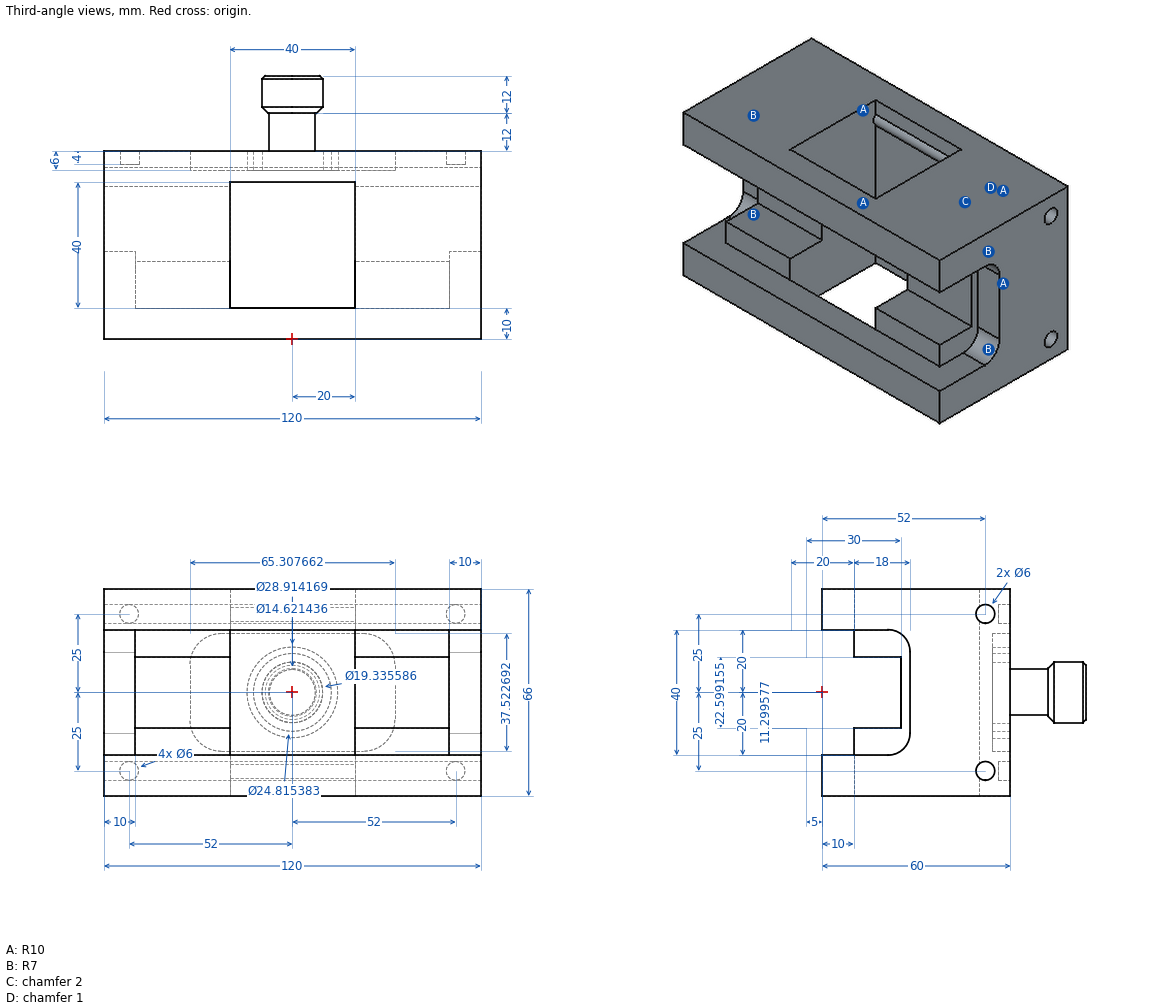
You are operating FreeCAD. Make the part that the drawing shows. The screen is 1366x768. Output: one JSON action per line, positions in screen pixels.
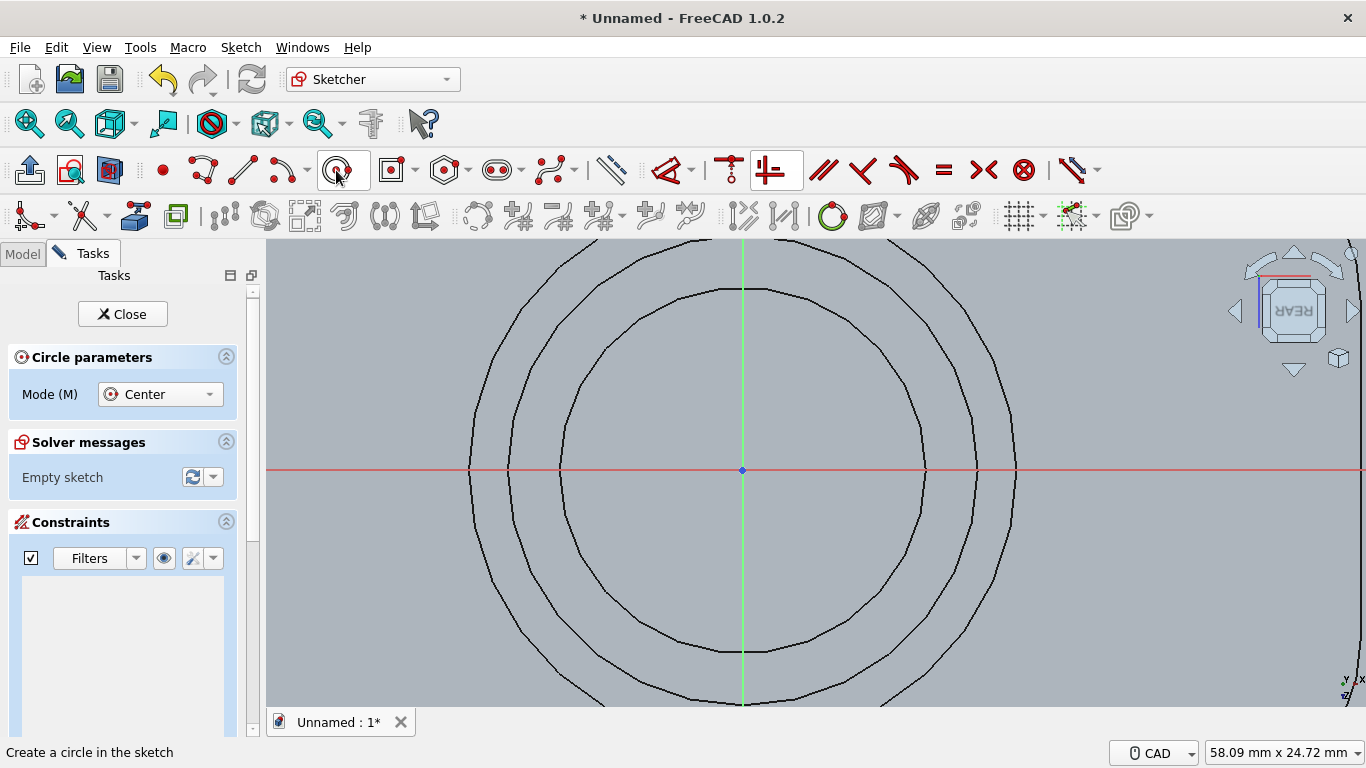
{"action": "left_click", "coordinate": [743, 470]}
{"action": "mouse_move", "coordinate": [841, 373]}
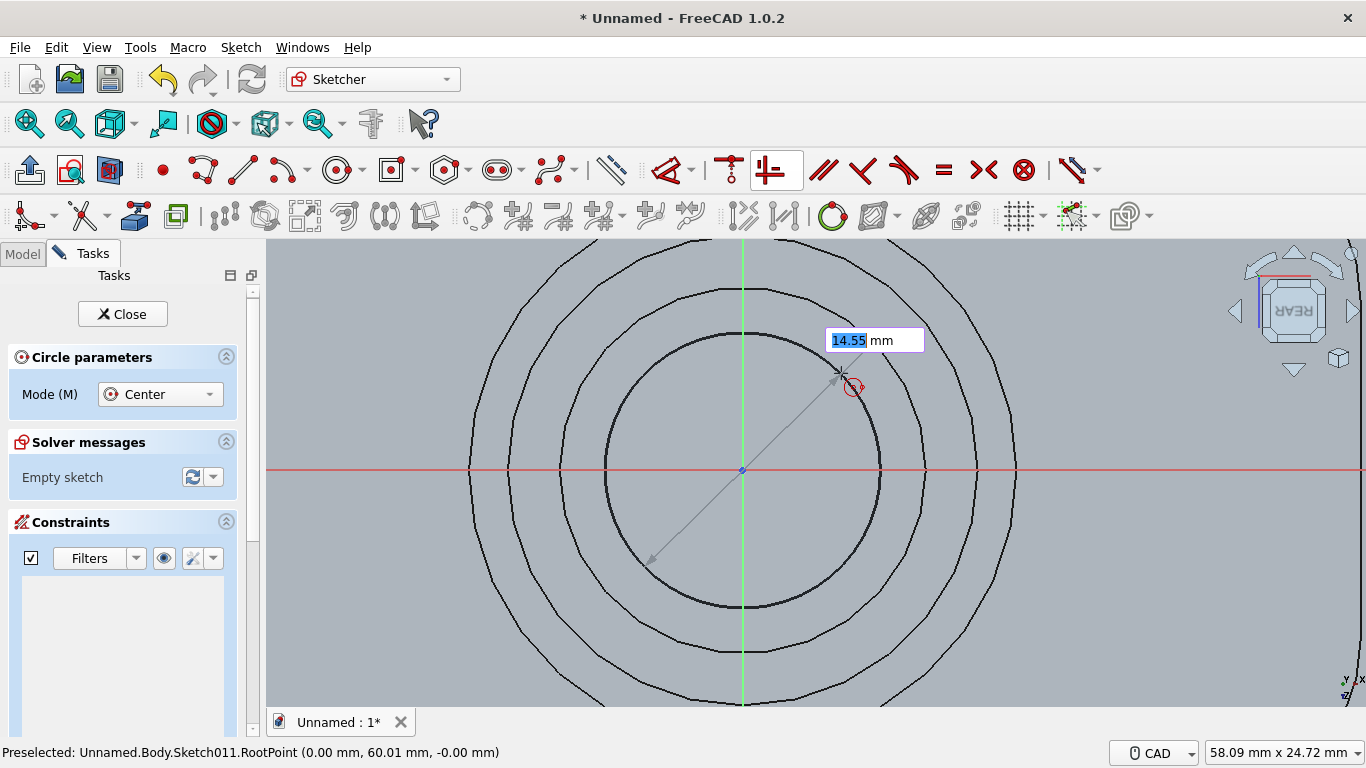
{"action": "type", "text": "14.621436"}
{"action": "key", "text": "Return"}
{"action": "key", "text": "Escape"}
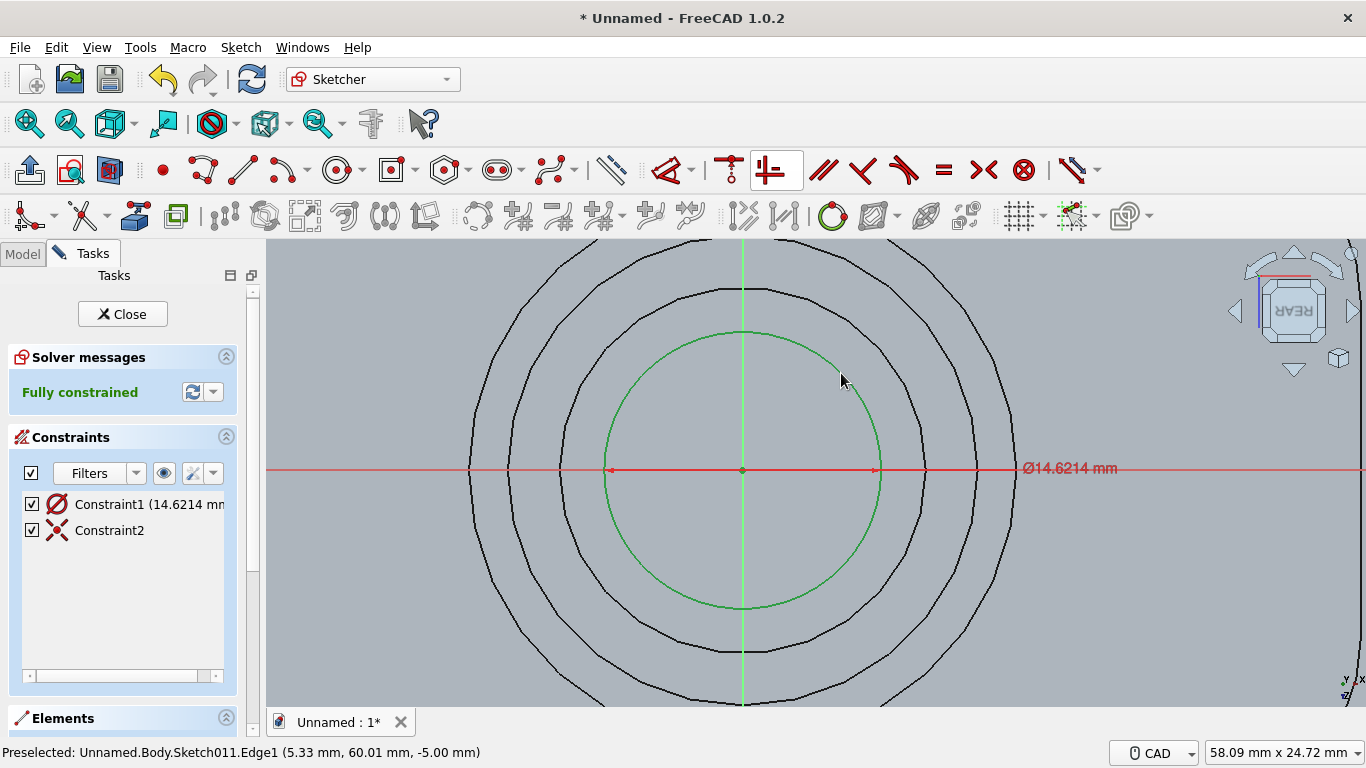
{"action": "left_click", "coordinate": [123, 314]}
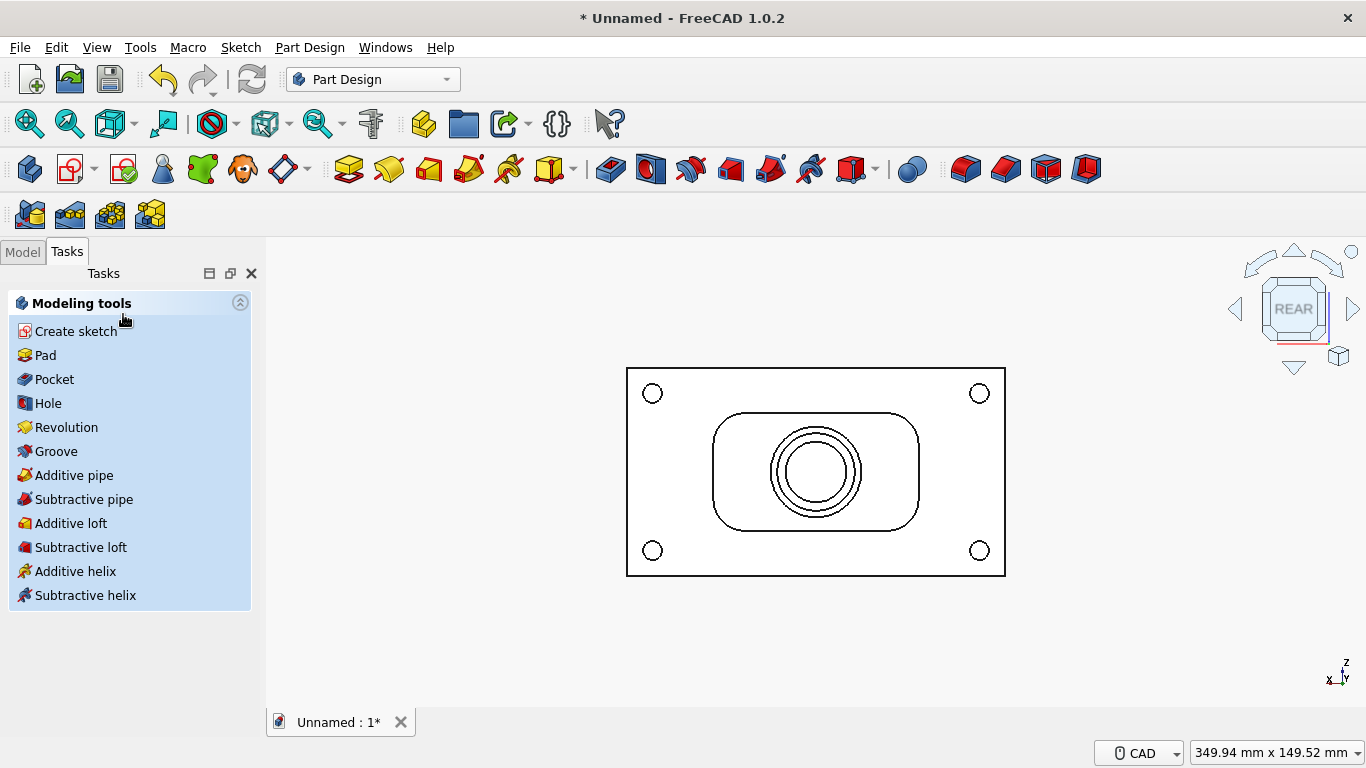
{"action": "left_click", "coordinate": [350, 170]}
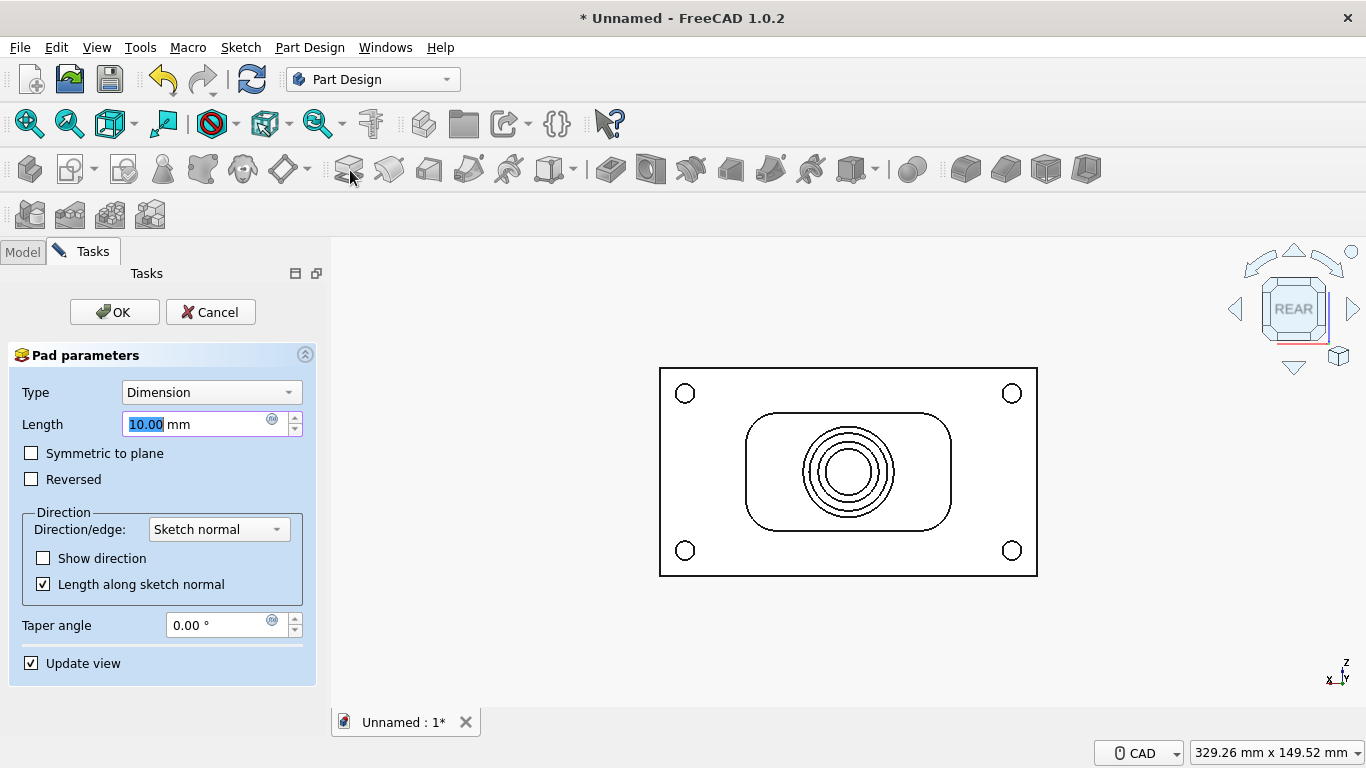
{"action": "type", "text": "12"}
{"action": "key", "text": "Tab"}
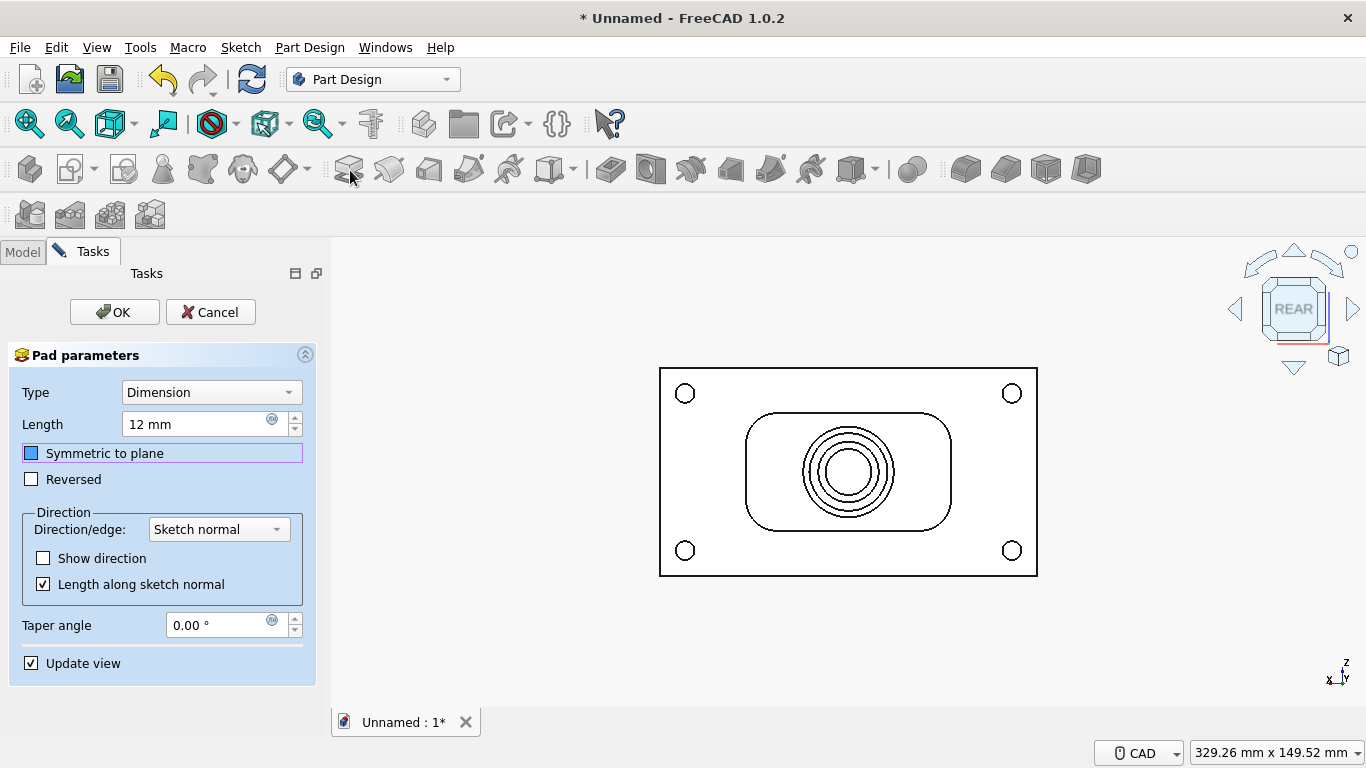
{"action": "left_click", "coordinate": [115, 312]}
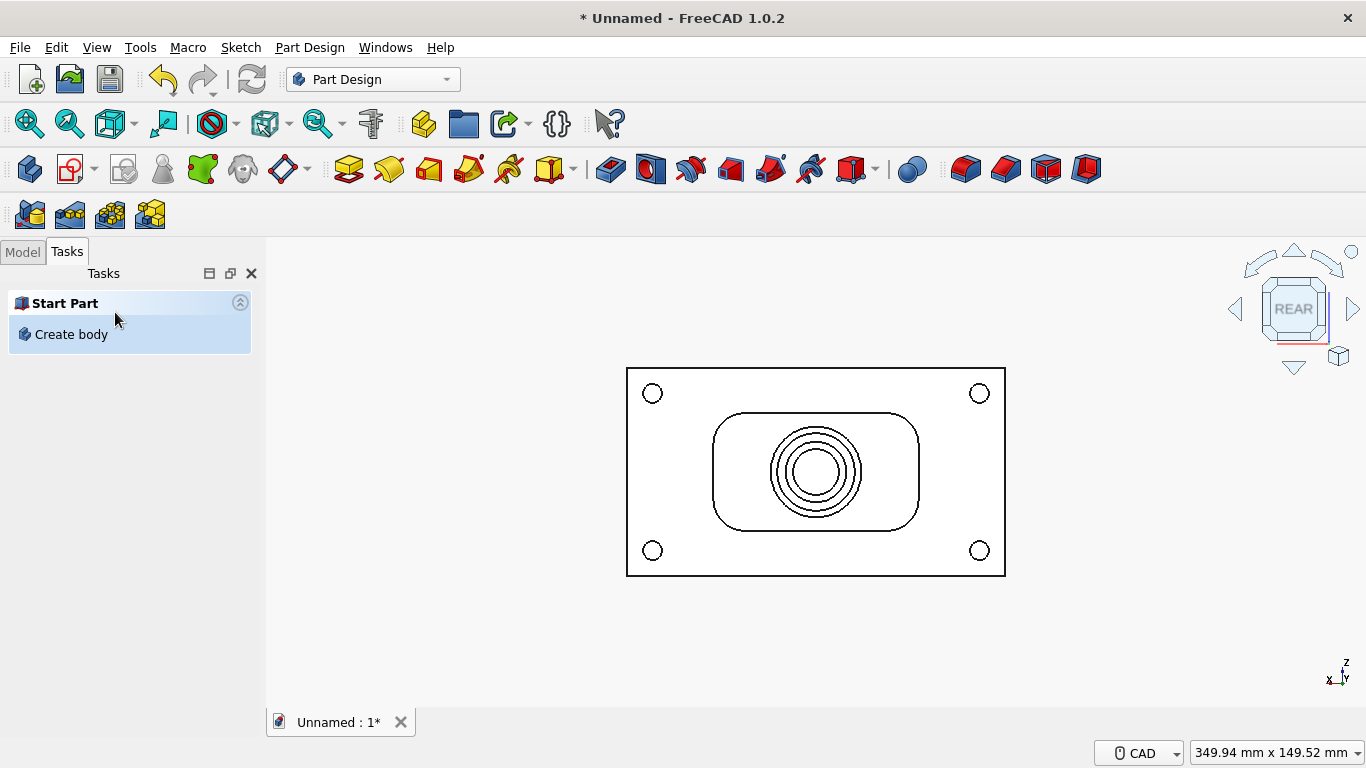
{"action": "left_click", "coordinate": [30, 124]}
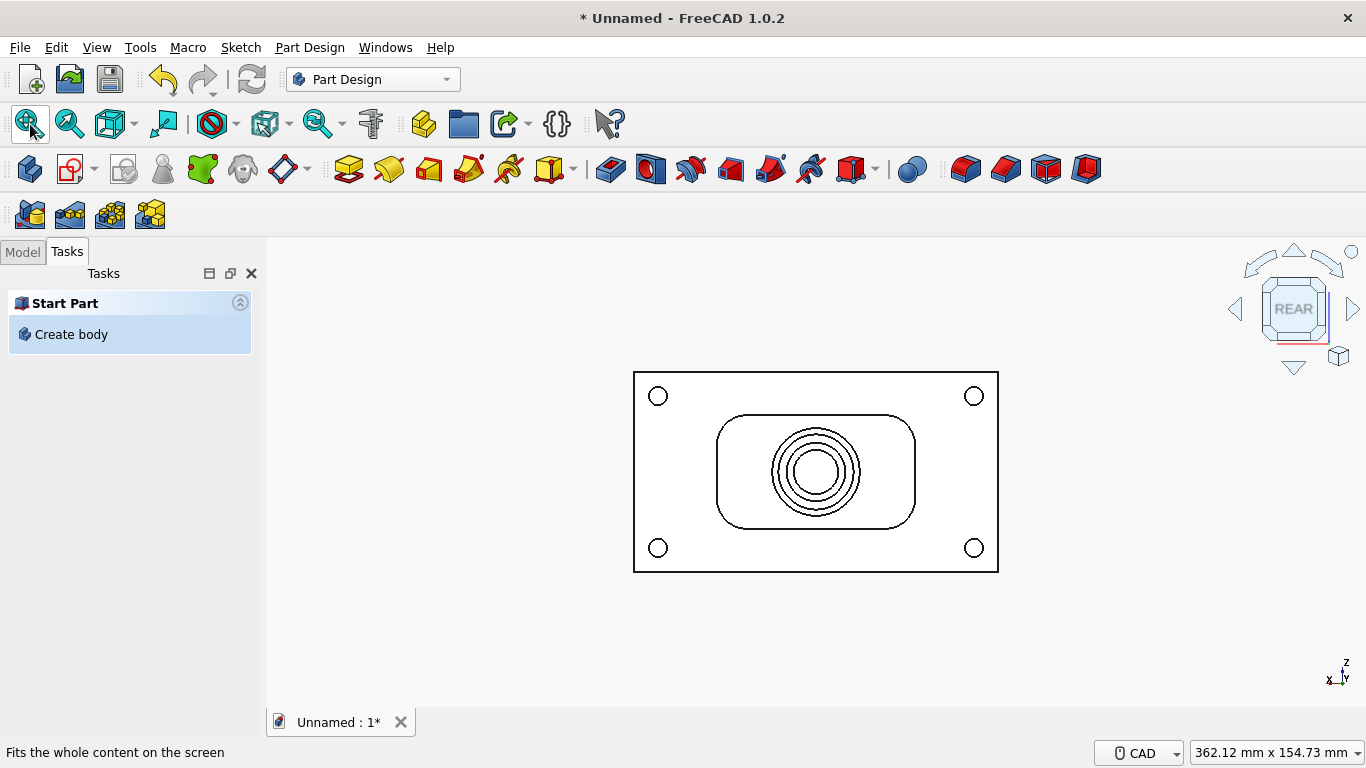
{"action": "left_click", "coordinate": [816, 471]}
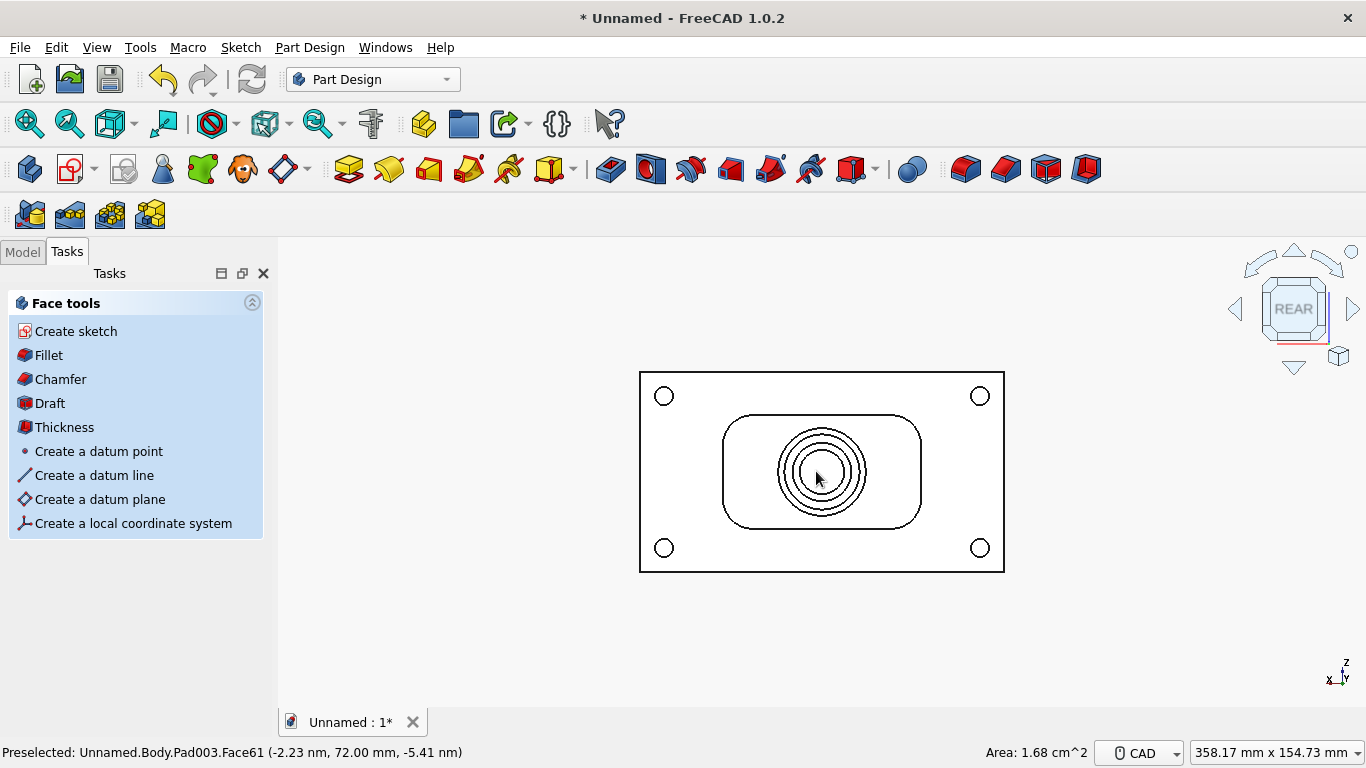
{"action": "left_click", "coordinate": [70, 170]}